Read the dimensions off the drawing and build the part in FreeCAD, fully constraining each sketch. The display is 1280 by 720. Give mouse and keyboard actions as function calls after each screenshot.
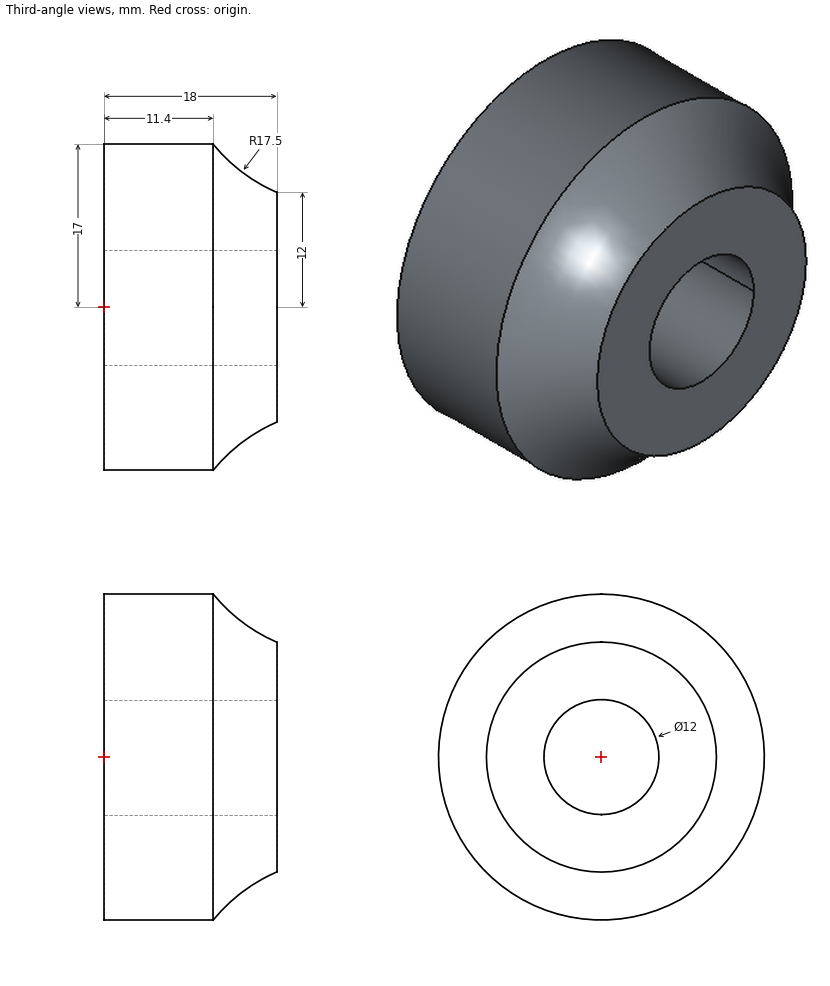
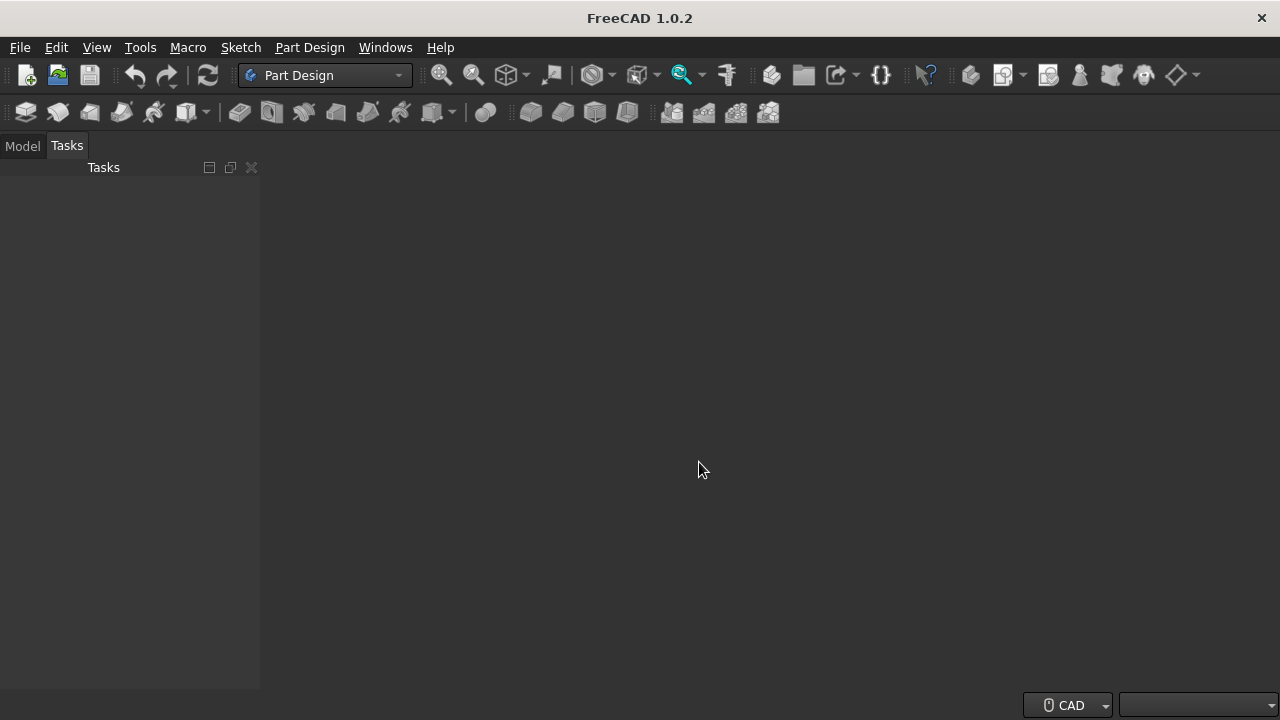
click(26, 76)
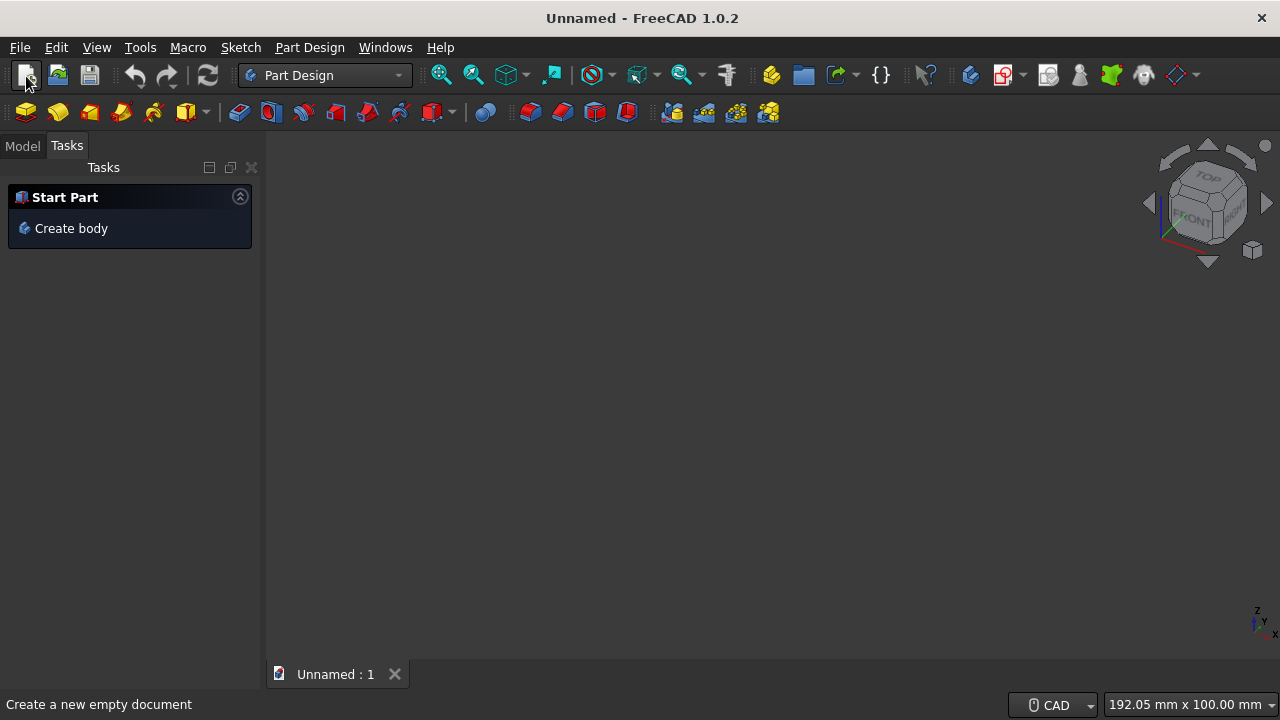
click(1004, 76)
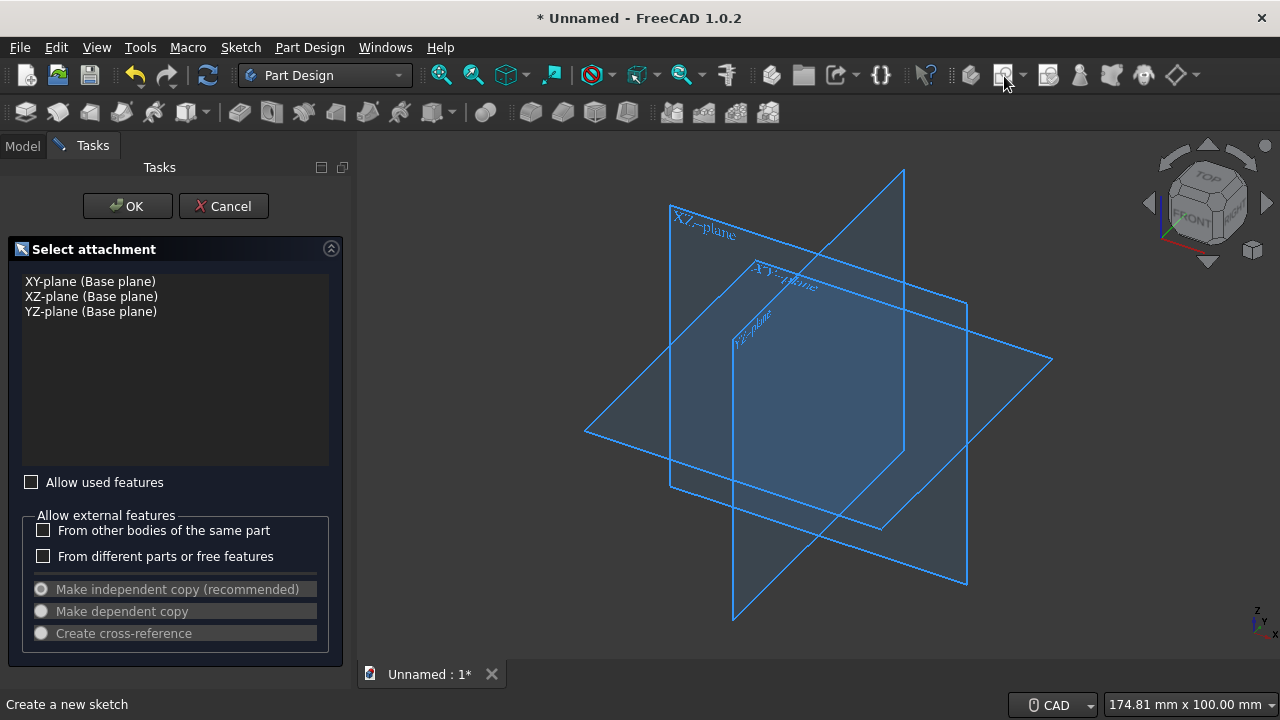
click(82, 282)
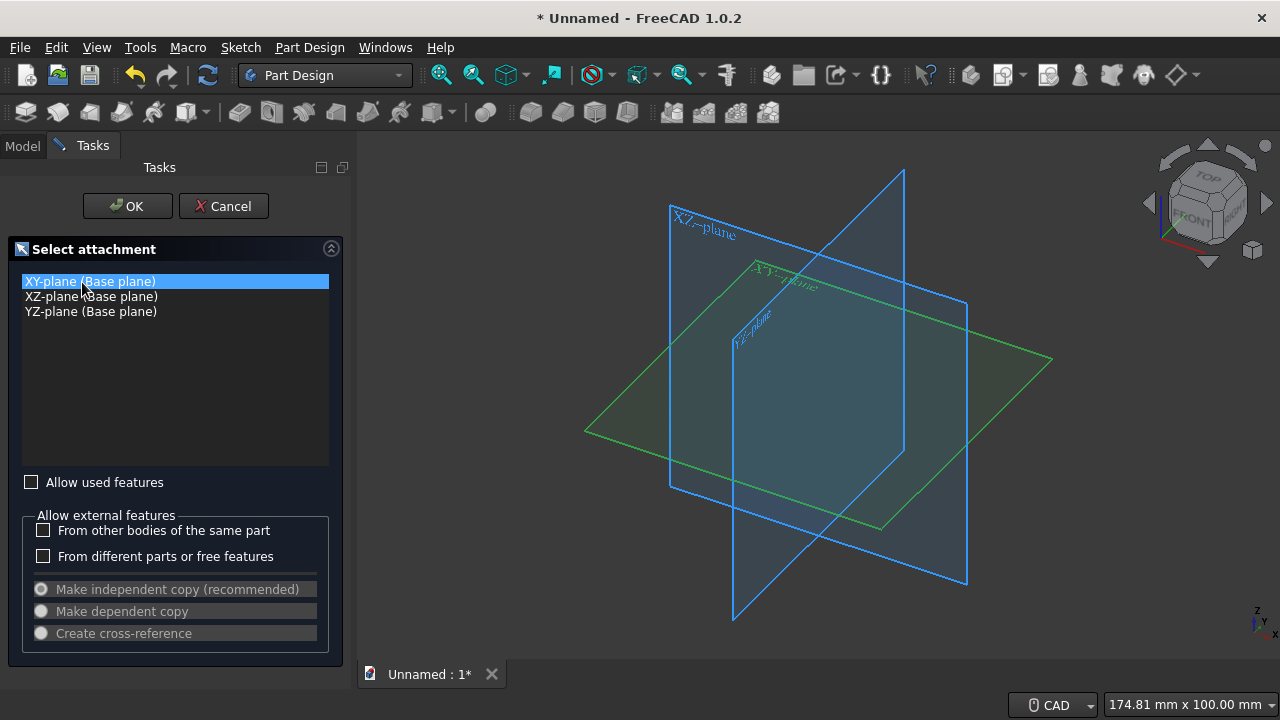
click(128, 206)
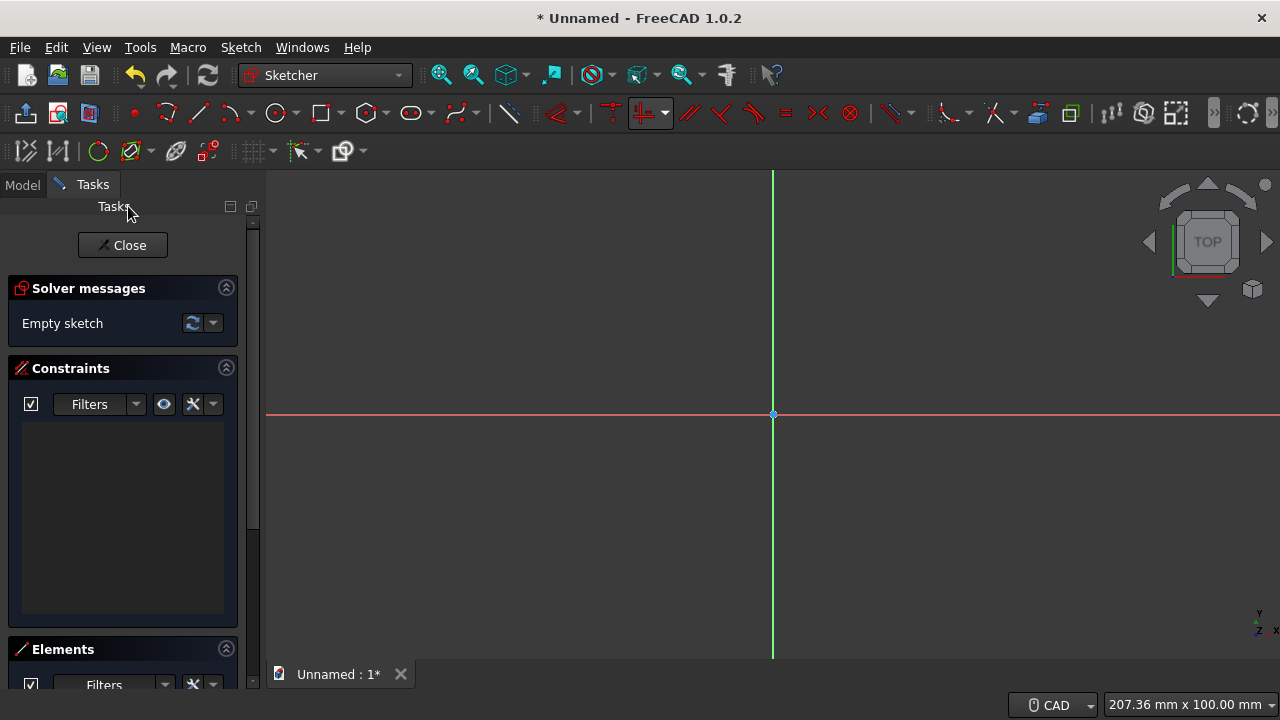
scroll(854, 359, up, 7)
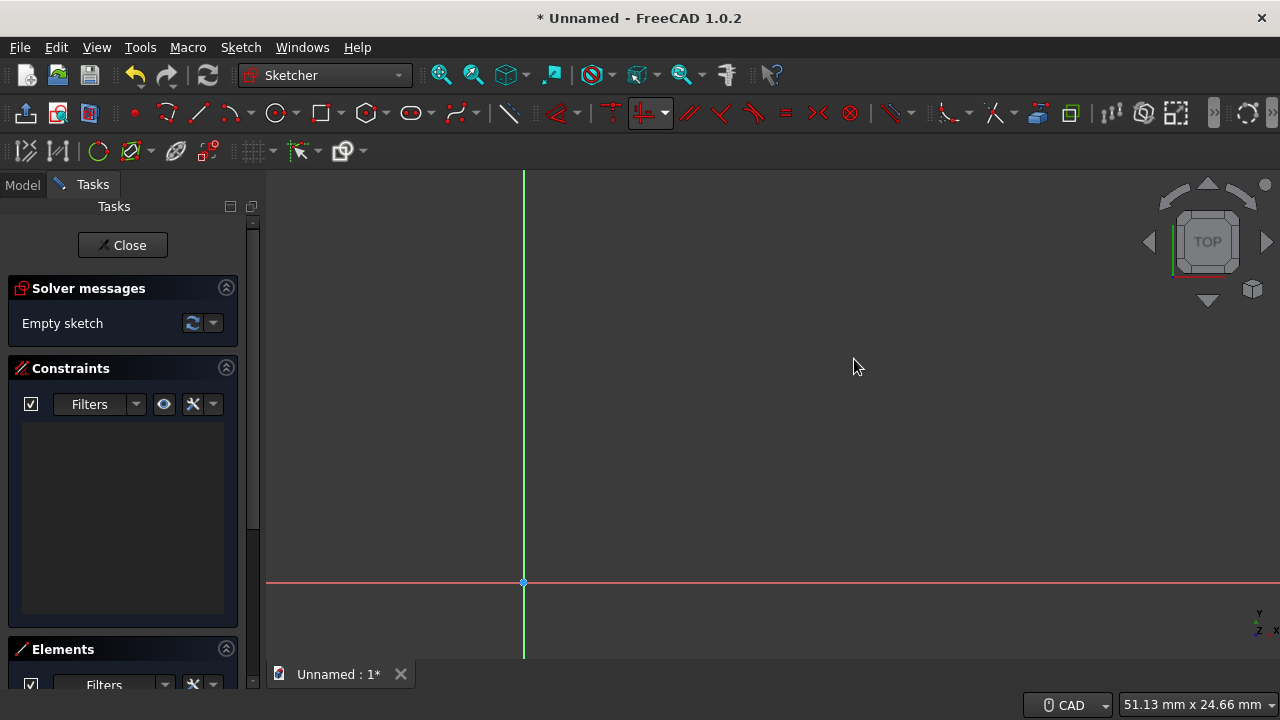
click(168, 114)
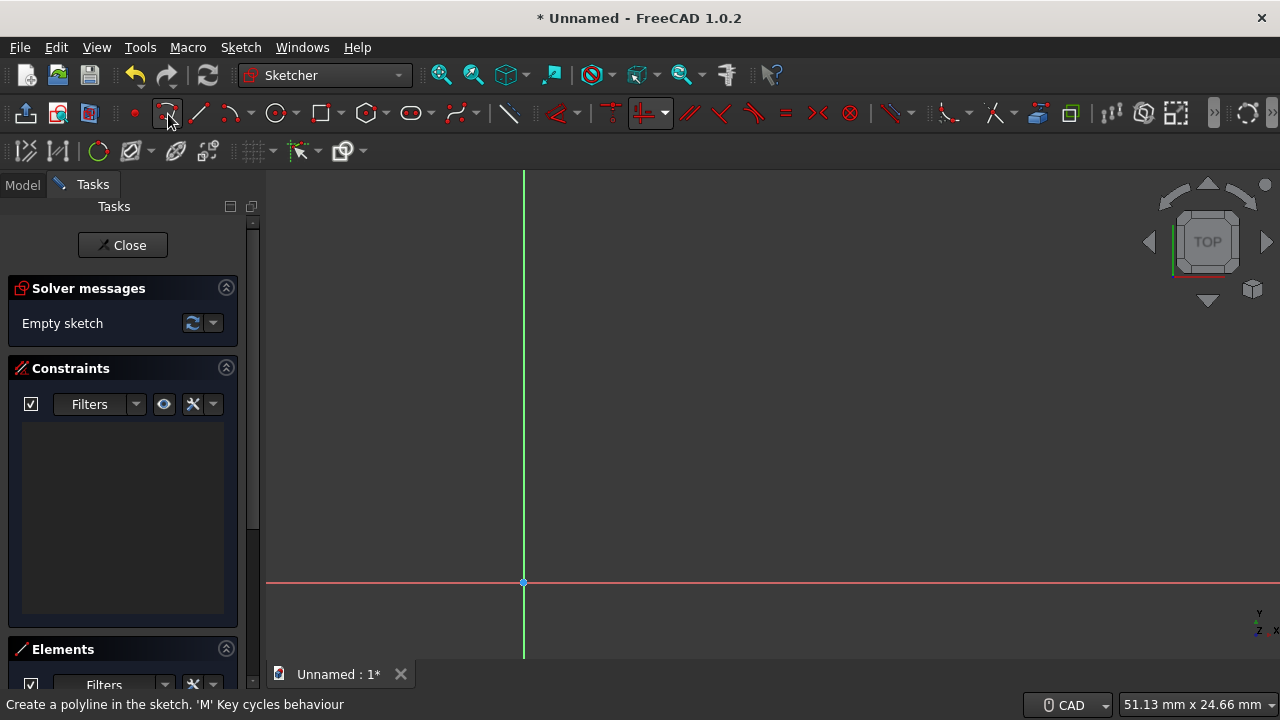
click(750, 246)
click(524, 246)
click(524, 583)
click(881, 574)
click(881, 345)
right_click(881, 345)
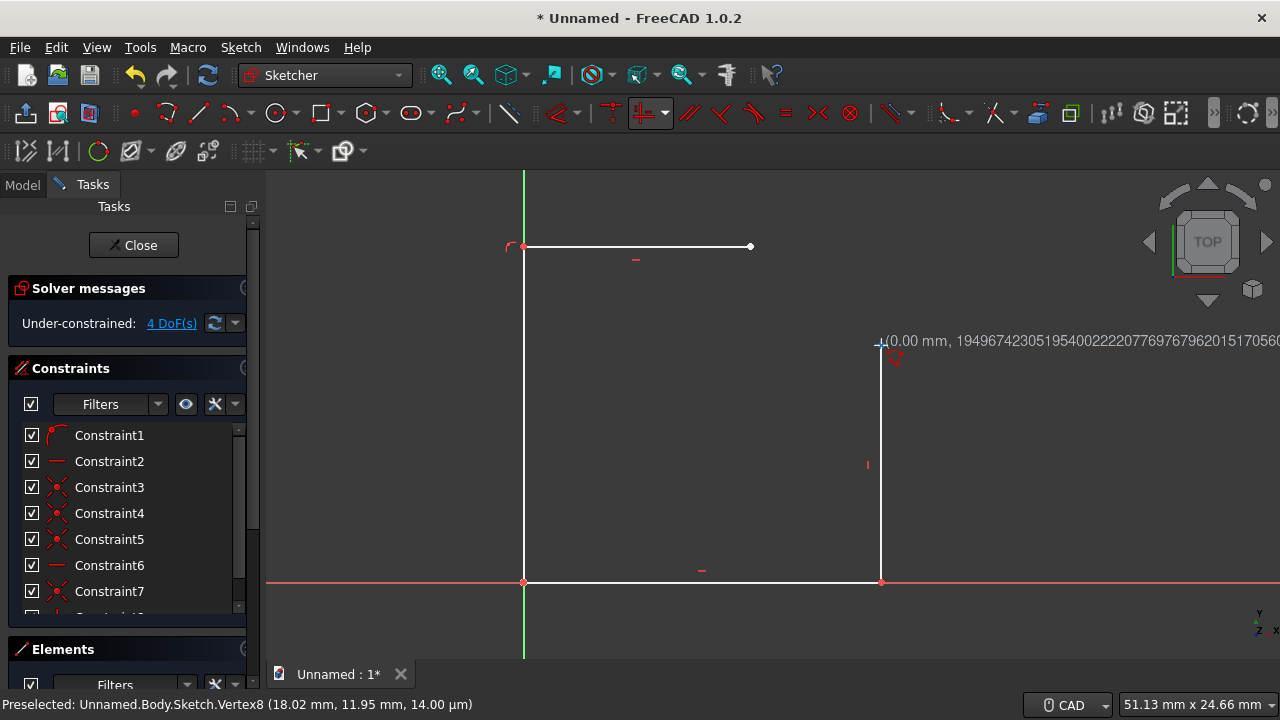
key(g)
key(3)
key(a)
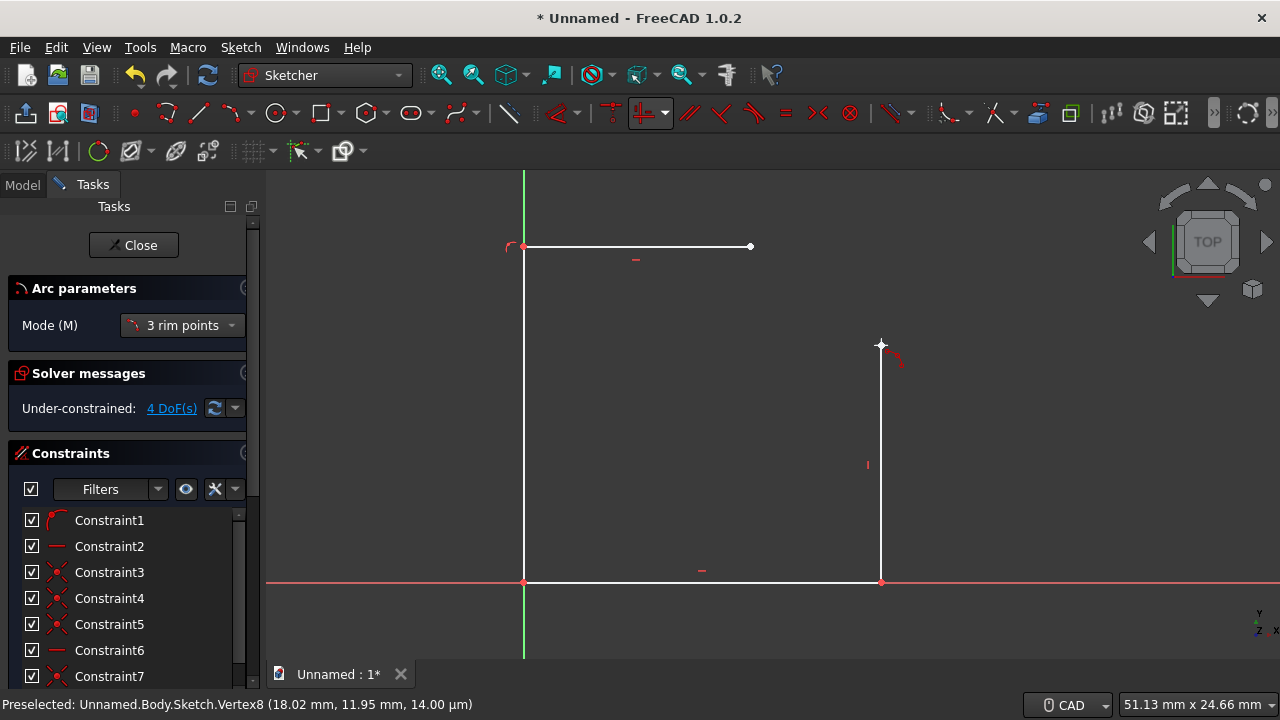
click(881, 346)
click(750, 247)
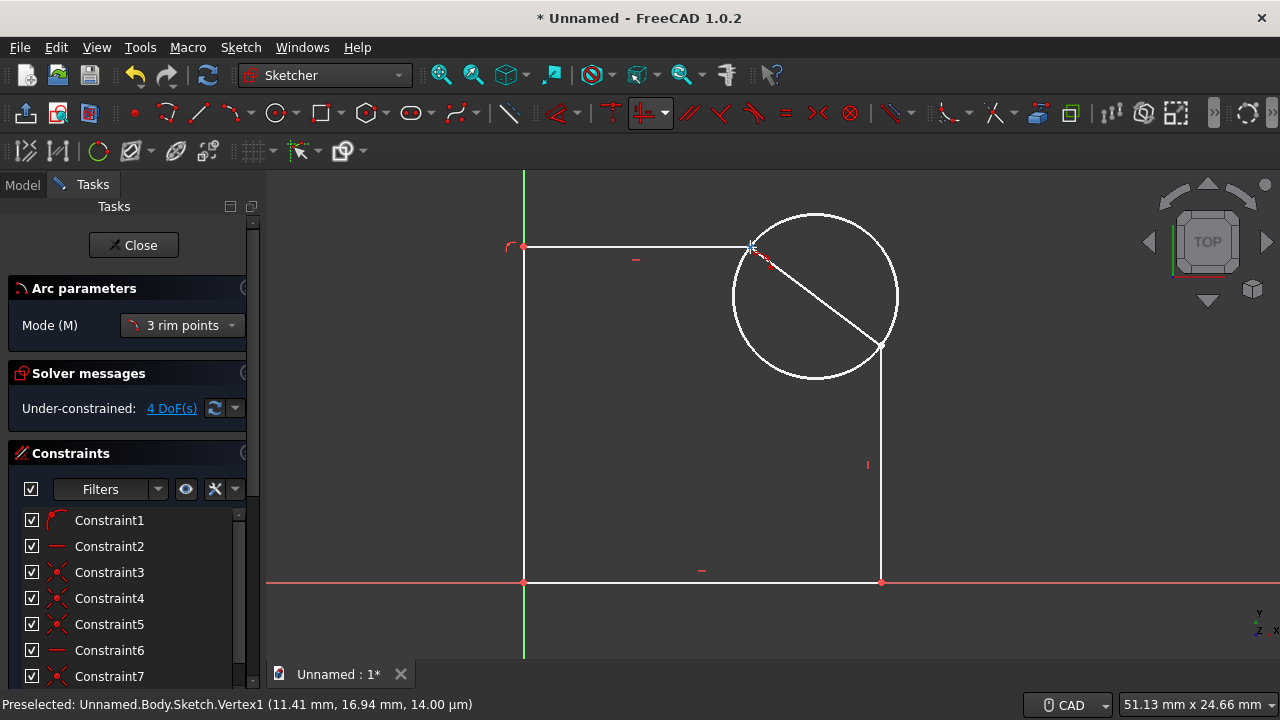
scroll(809, 303, up, 3)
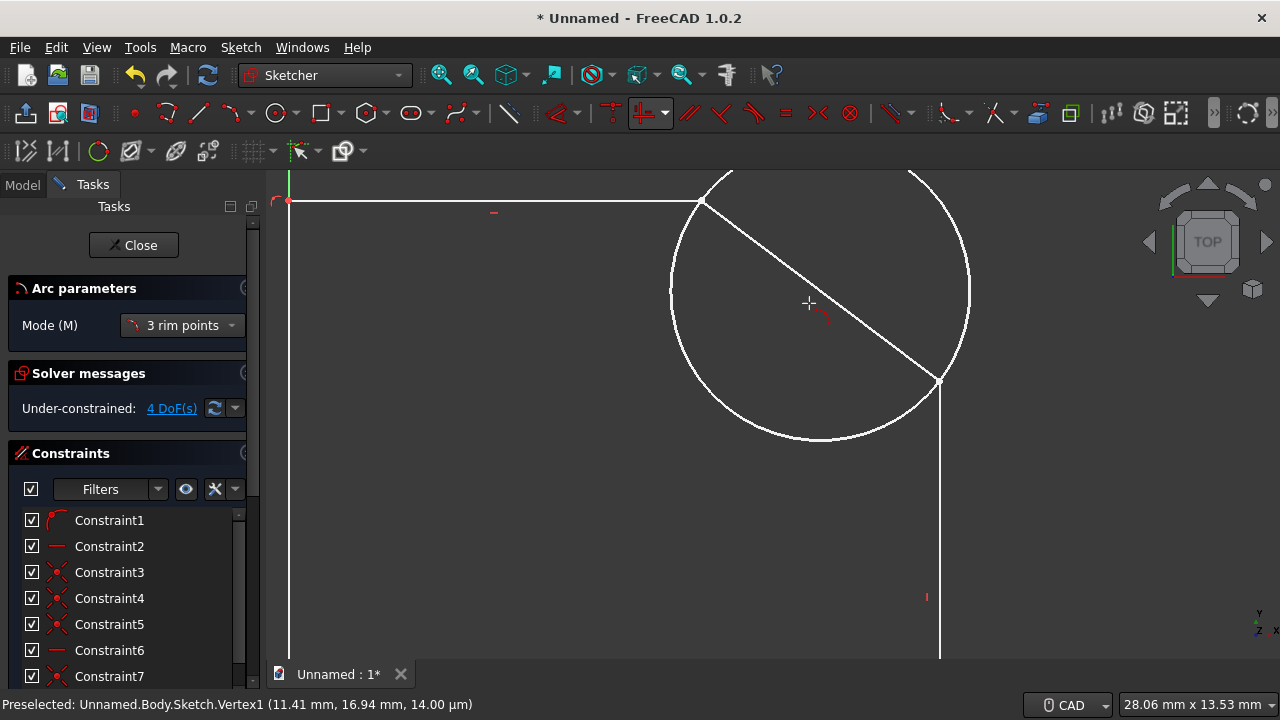
click(809, 303)
key(Escape)